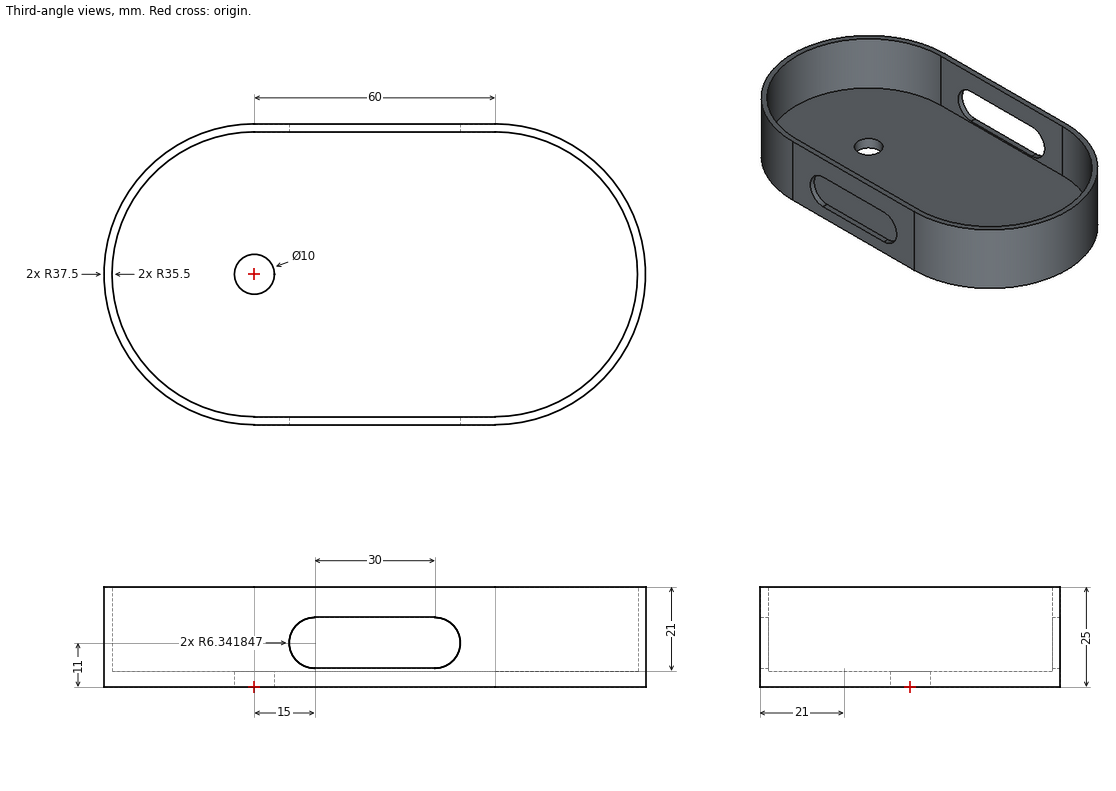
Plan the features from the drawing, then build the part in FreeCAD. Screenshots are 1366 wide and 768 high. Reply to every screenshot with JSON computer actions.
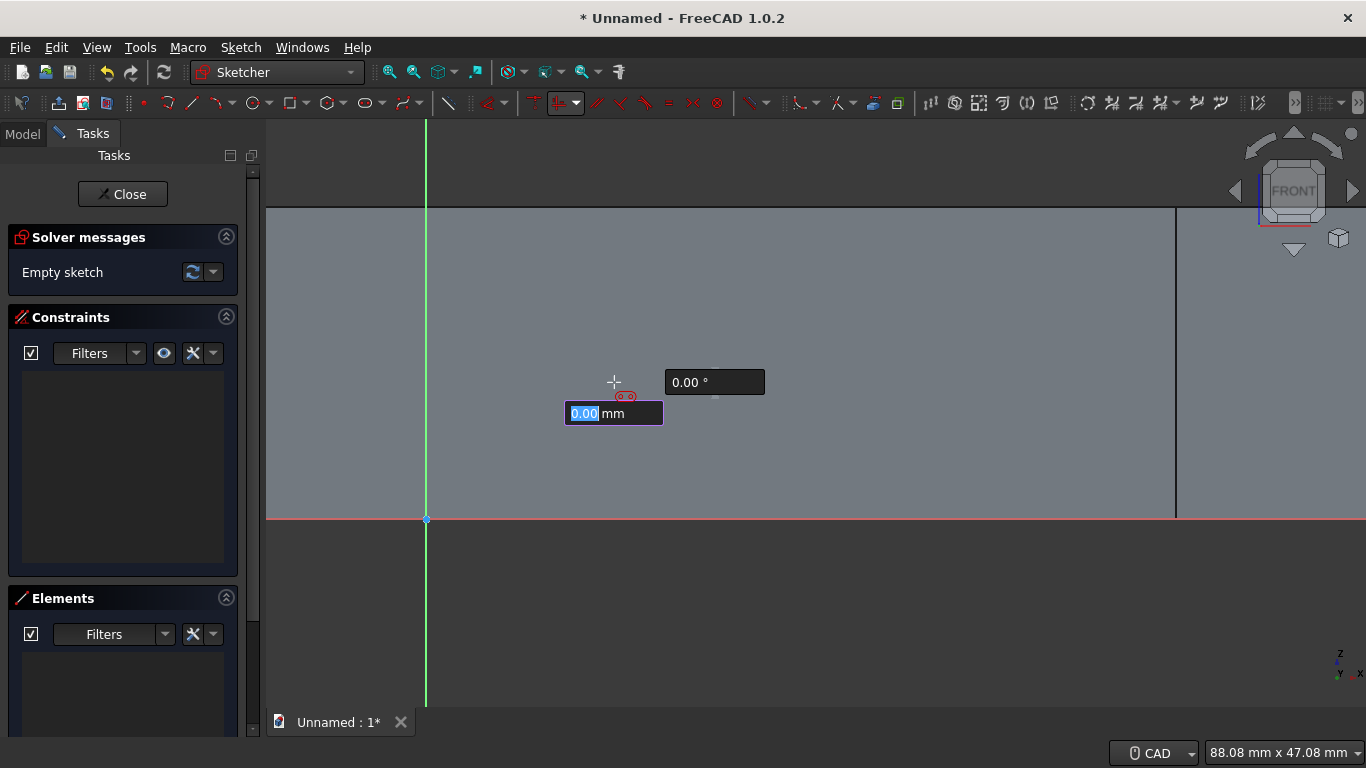
{"action": "left_click", "coordinate": [988, 382]}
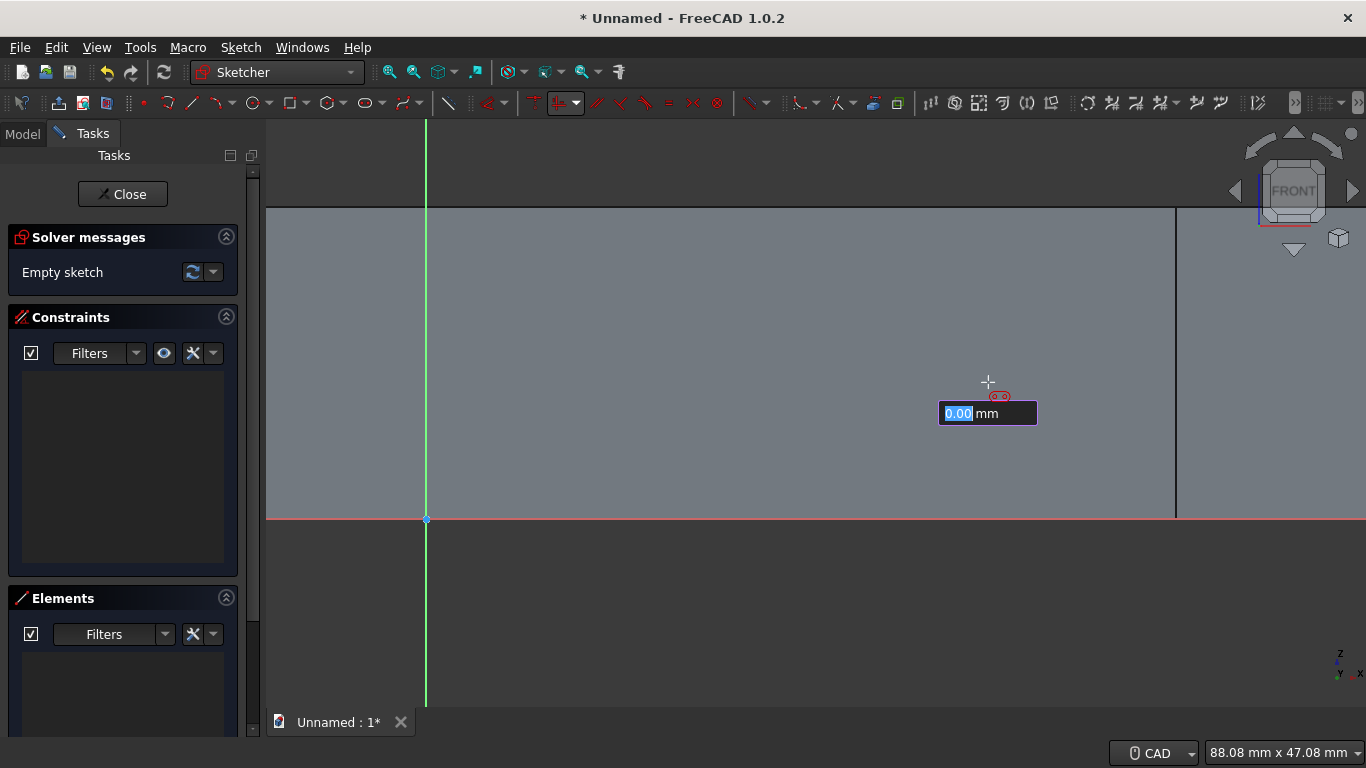
{"action": "left_click", "coordinate": [801, 303]}
{"action": "key", "text": "Escape"}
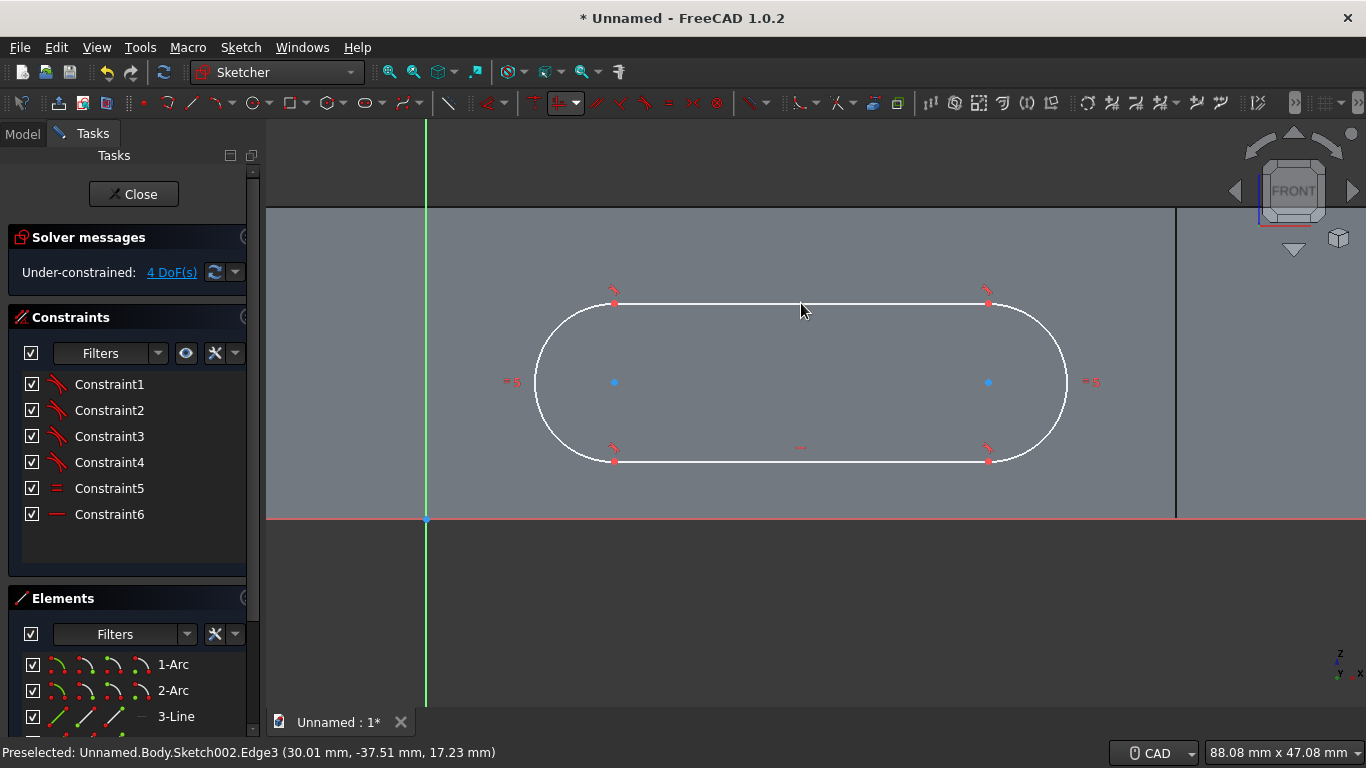
{"action": "left_click", "coordinate": [488, 104]}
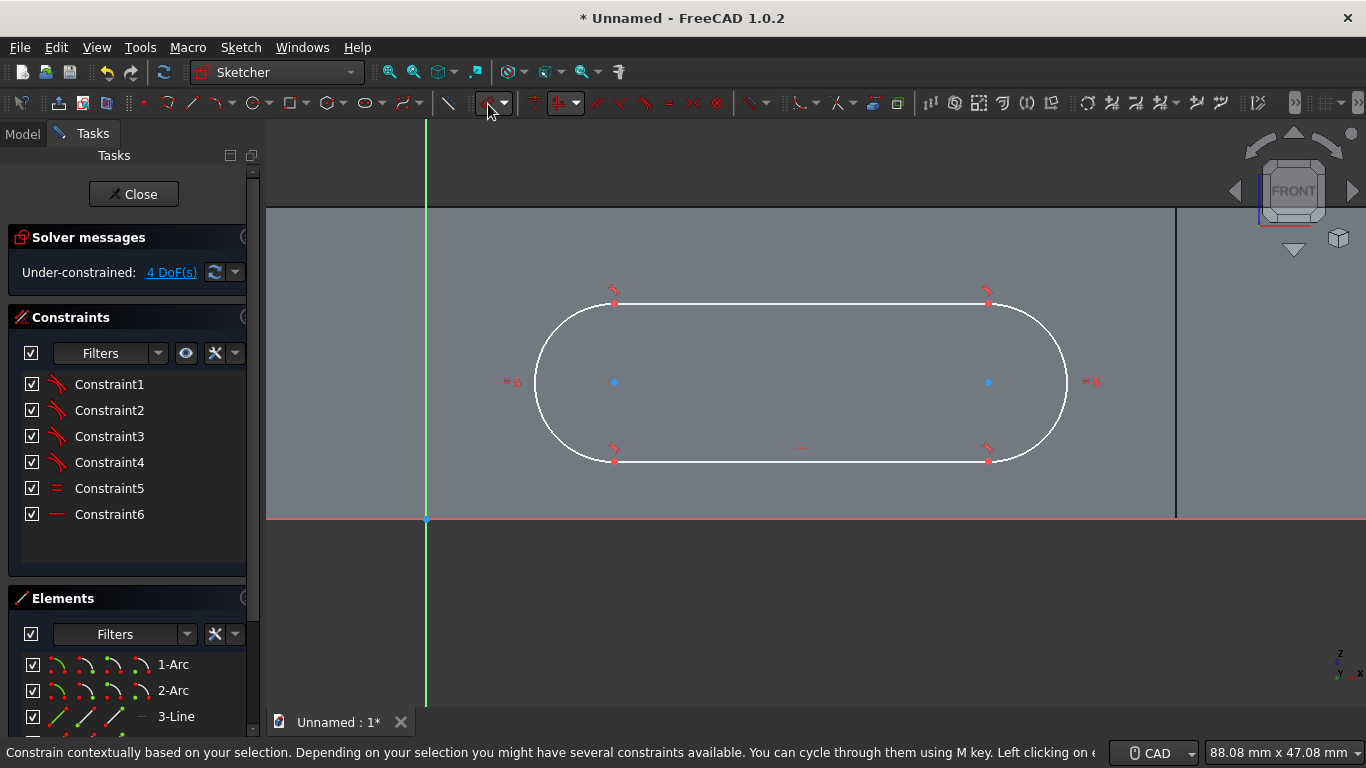
{"action": "left_click", "coordinate": [550, 337]}
{"action": "left_click", "coordinate": [524, 318]}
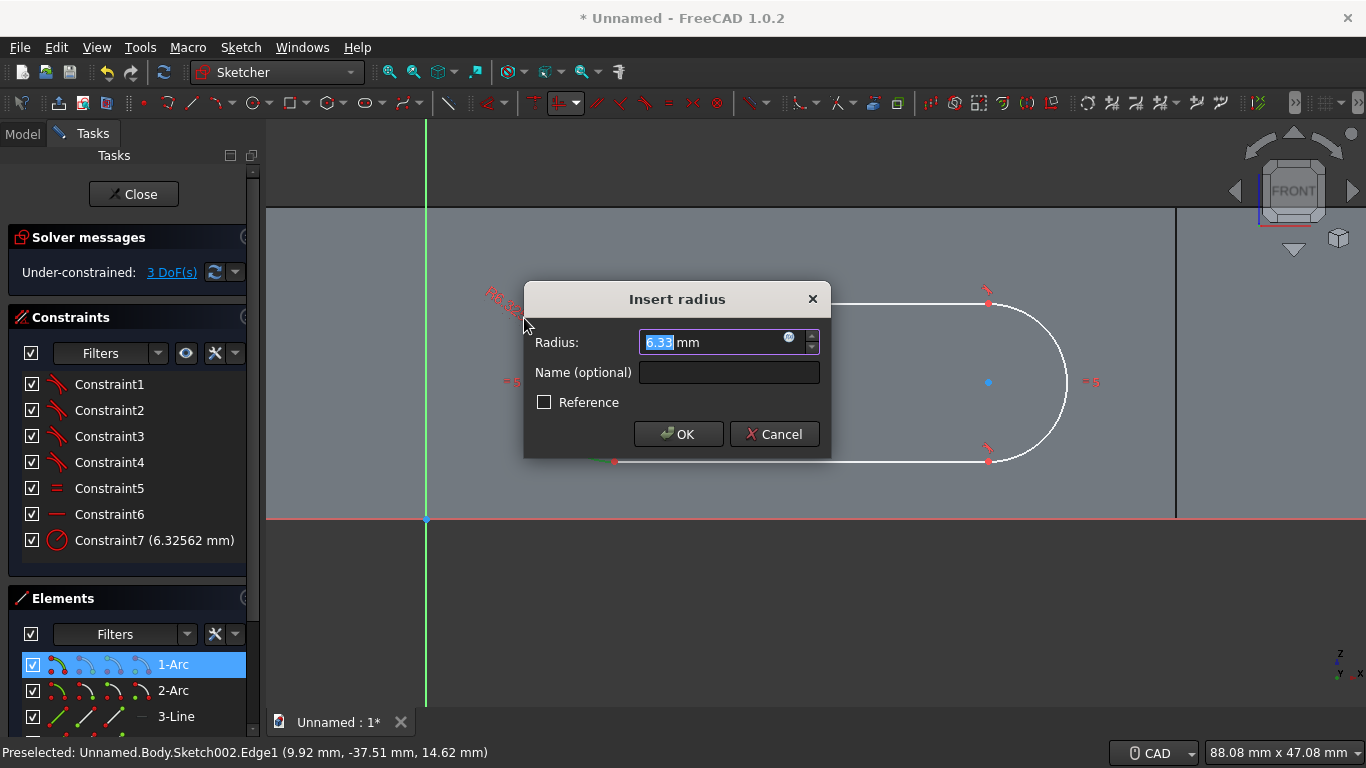
{"action": "type", "text": "6.341847"}
{"action": "key", "text": "Return"}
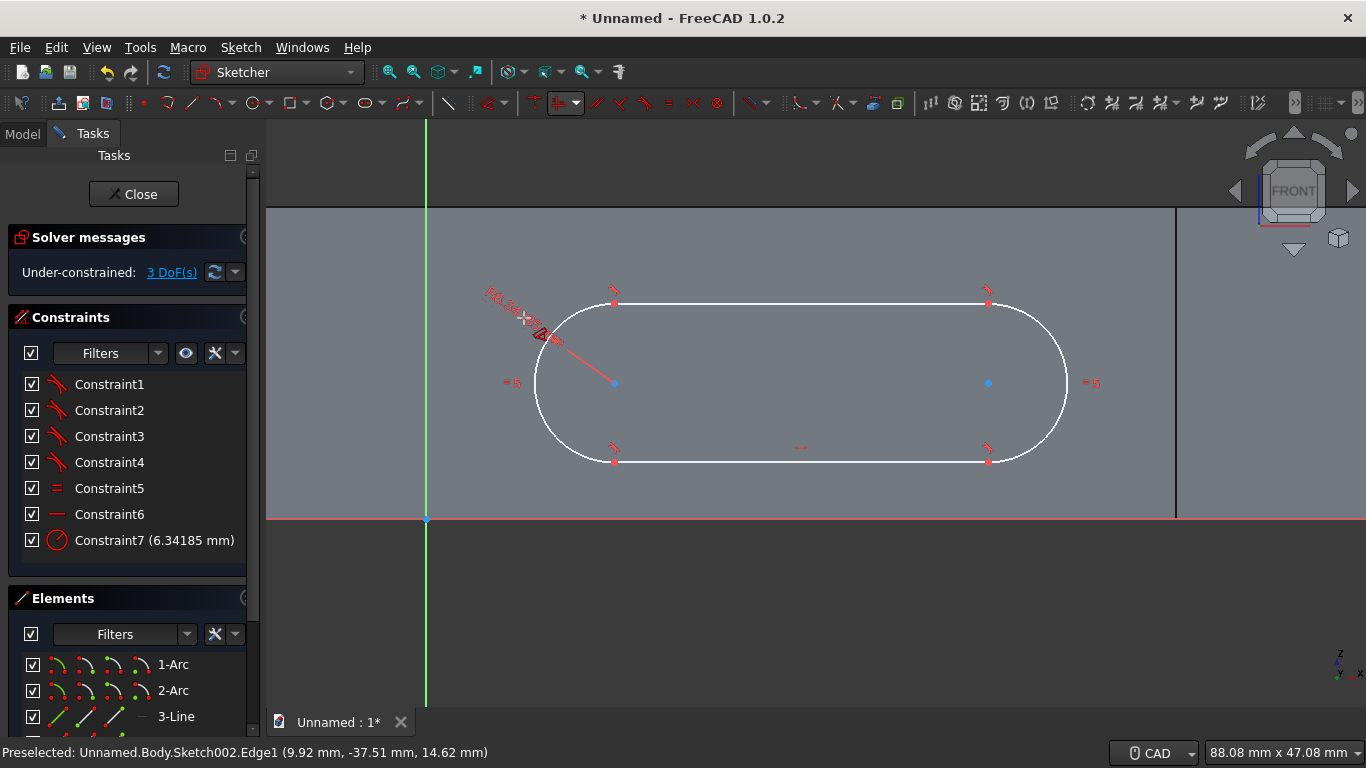
{"action": "left_click", "coordinate": [726, 304]}
{"action": "left_click", "coordinate": [801, 270]}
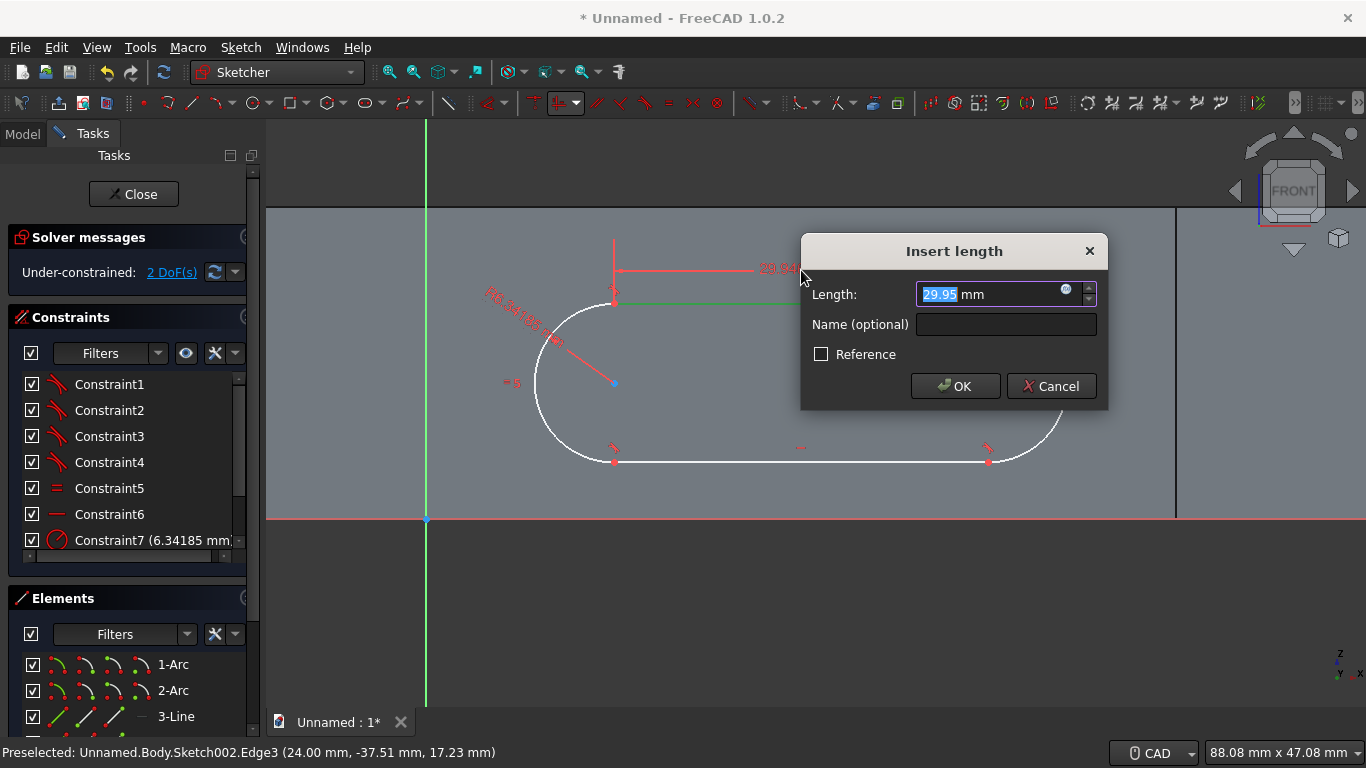
{"action": "type", "text": "30"}
{"action": "key", "text": "Return"}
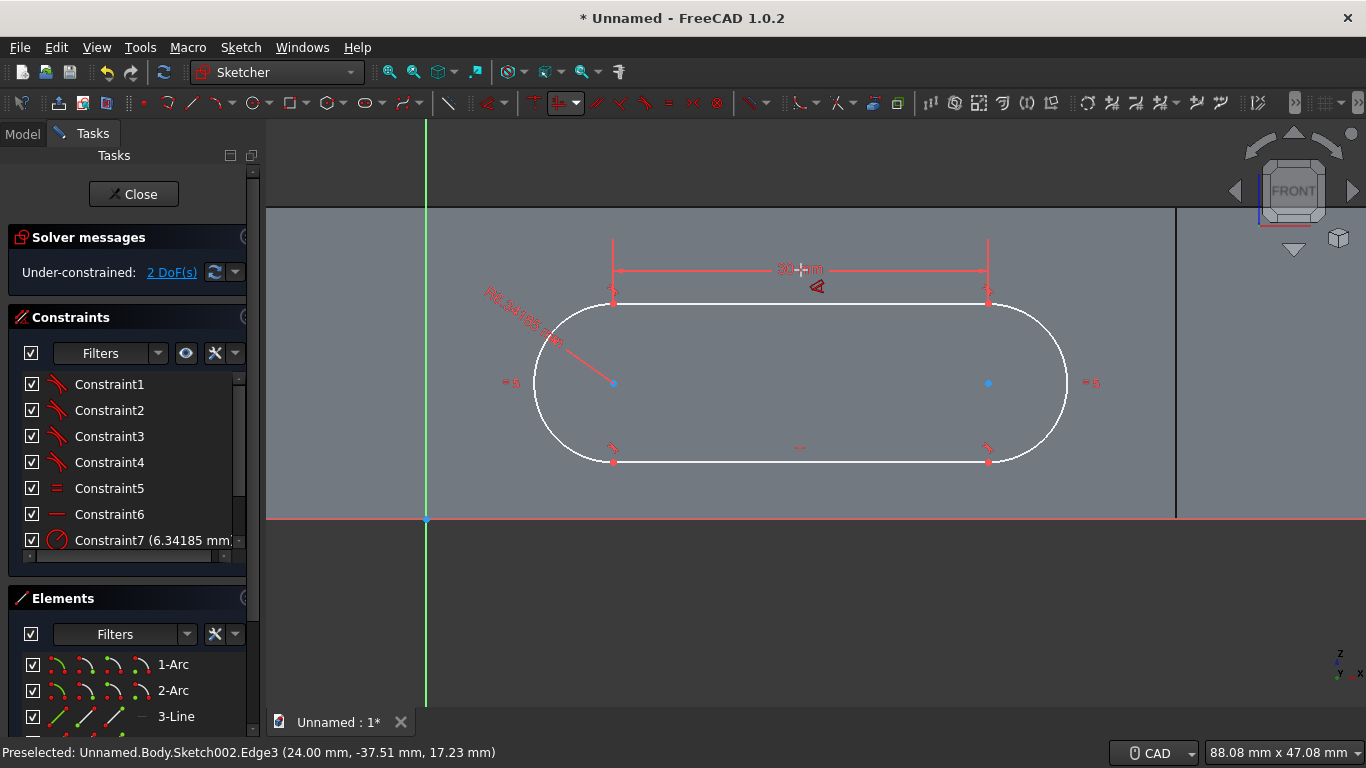
{"action": "left_click", "coordinate": [613, 304]}
{"action": "left_click", "coordinate": [520, 553]}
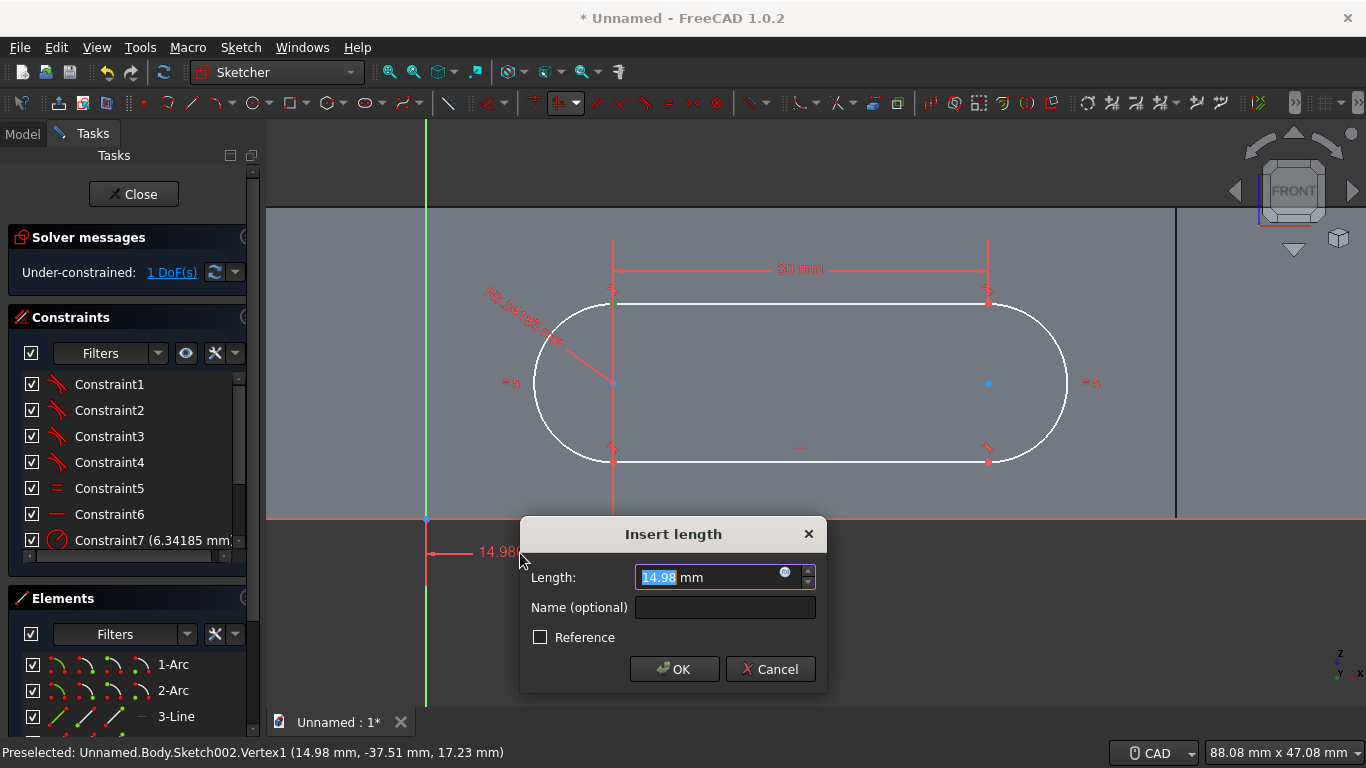
{"action": "type", "text": "15"}
{"action": "key", "text": "Return"}